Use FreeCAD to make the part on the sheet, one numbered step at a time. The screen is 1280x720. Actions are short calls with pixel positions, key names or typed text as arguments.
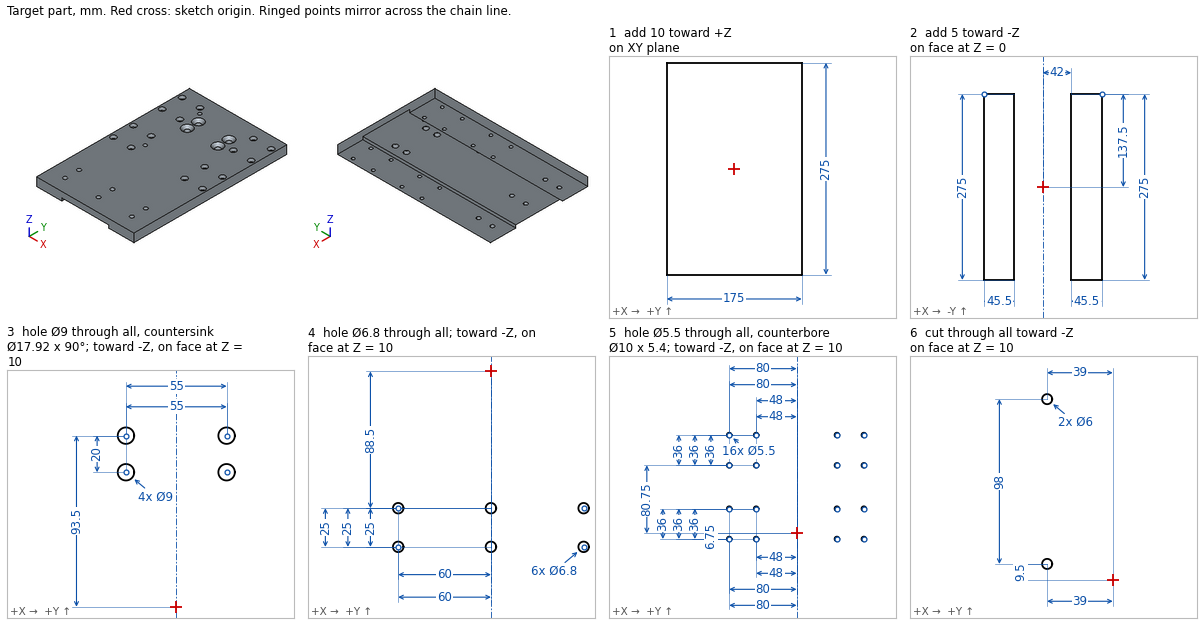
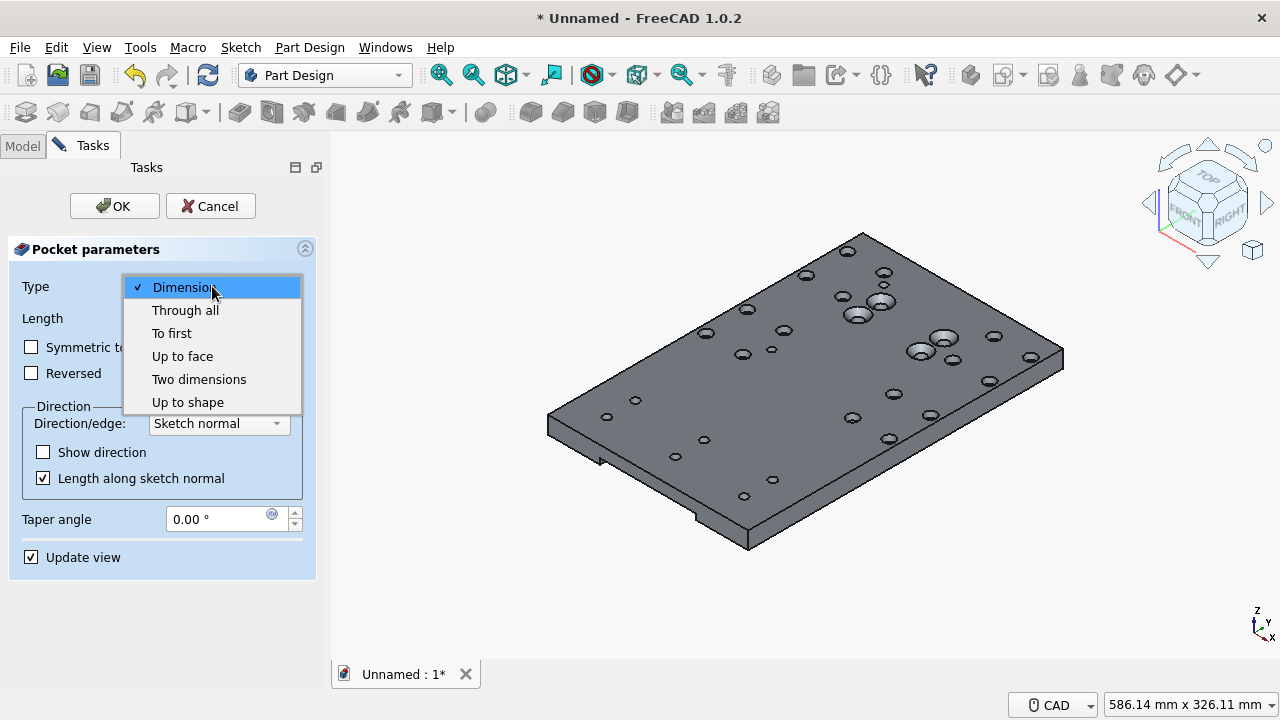
click(212, 310)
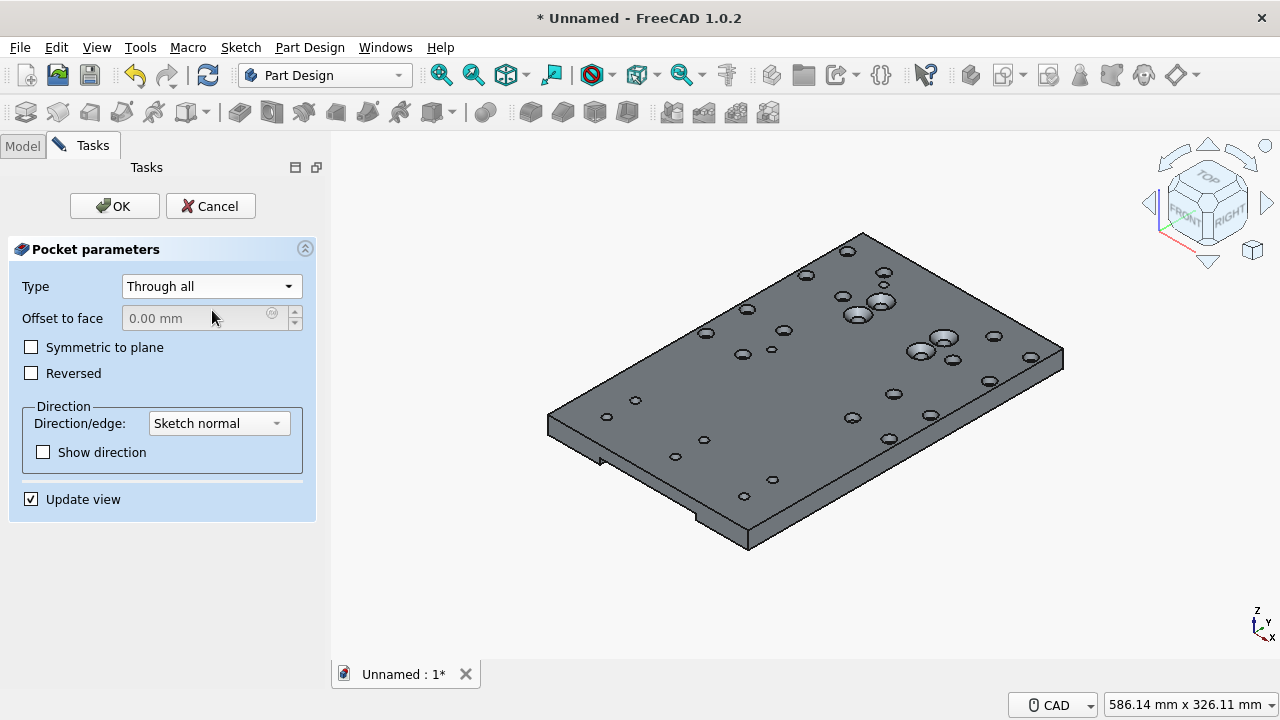
click(115, 206)